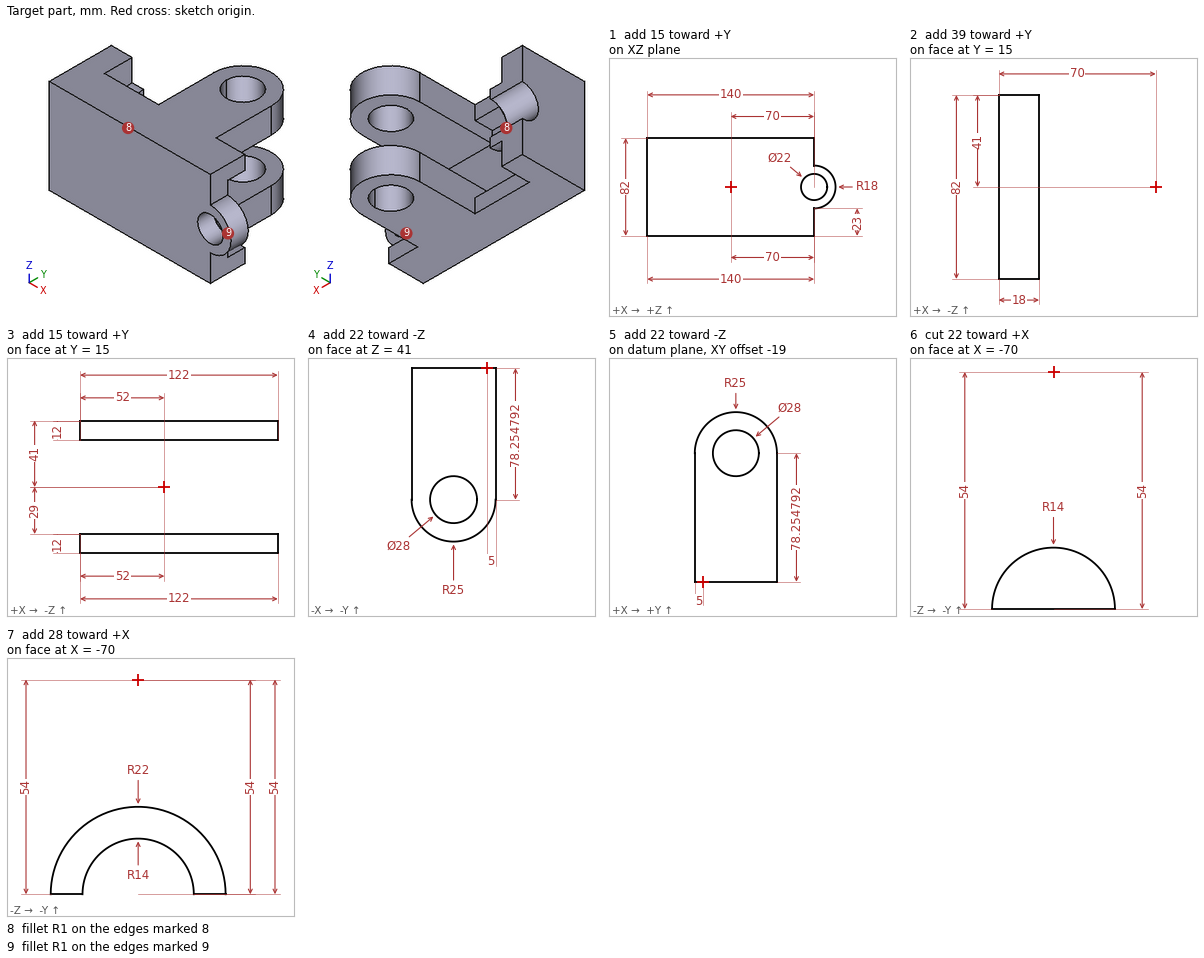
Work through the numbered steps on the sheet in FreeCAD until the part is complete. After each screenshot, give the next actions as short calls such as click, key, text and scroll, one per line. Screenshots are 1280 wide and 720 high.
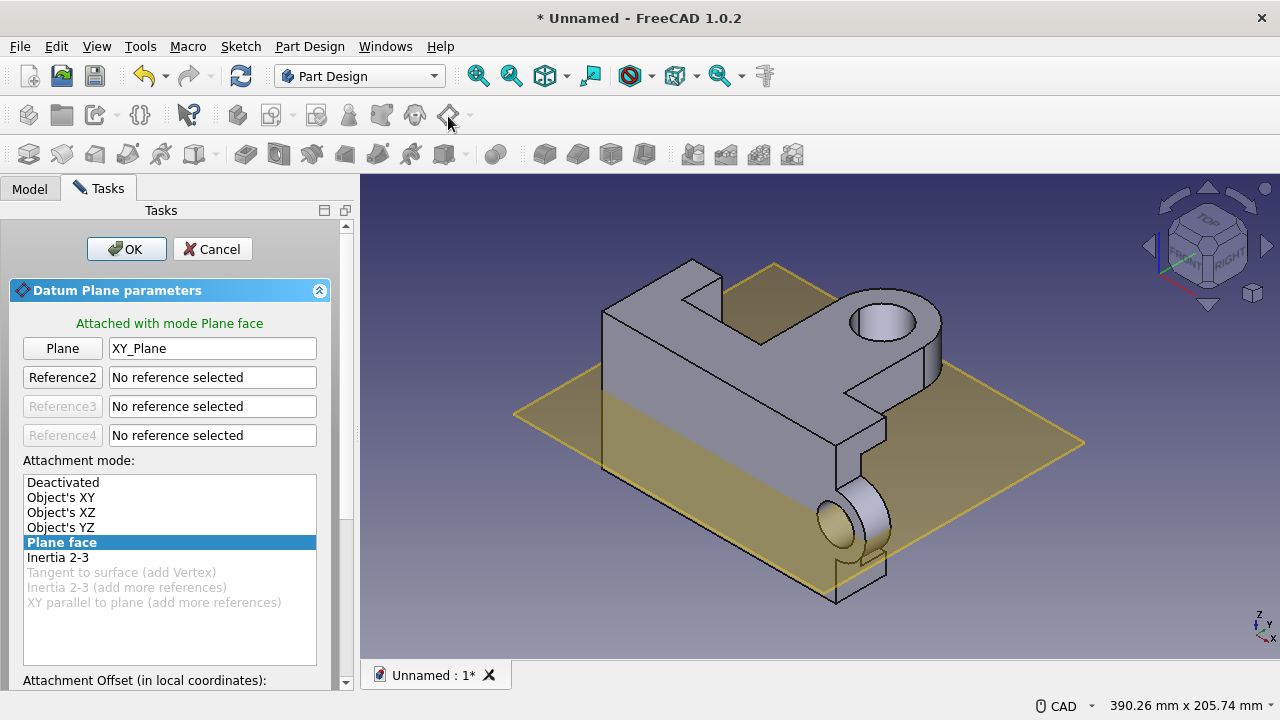
scroll(346, 455, down, 3)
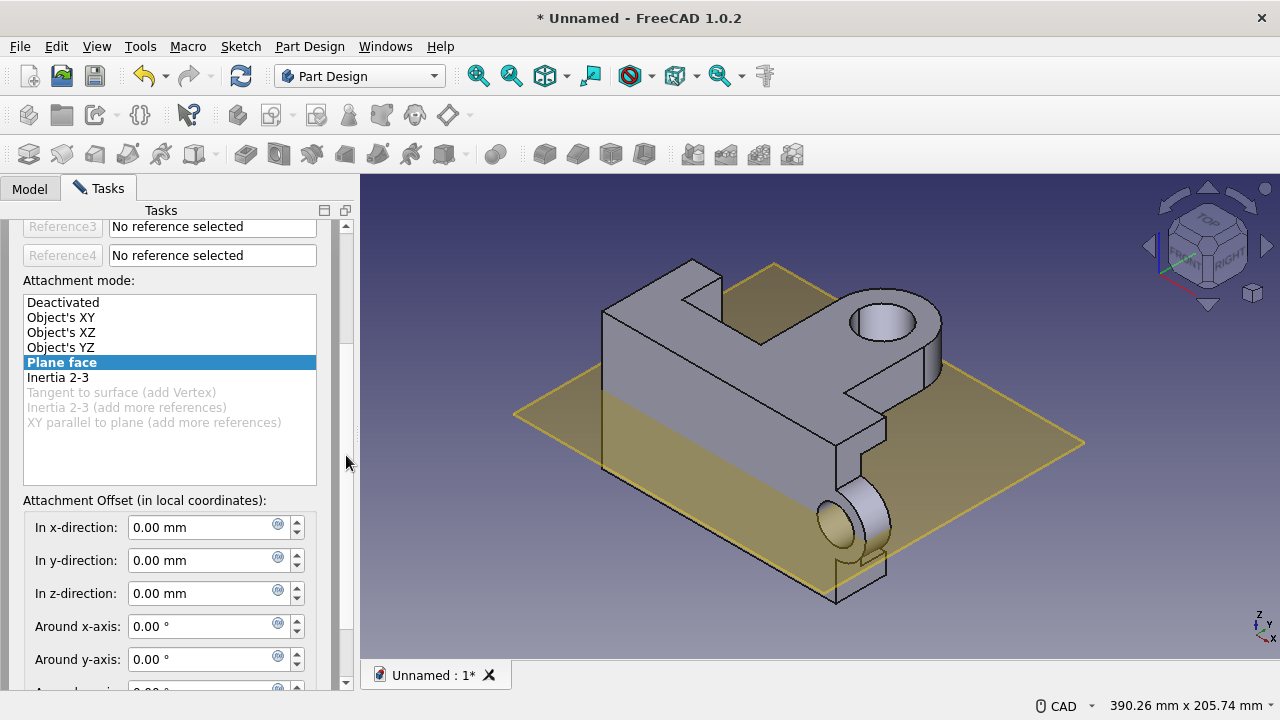
triple_click(210, 594)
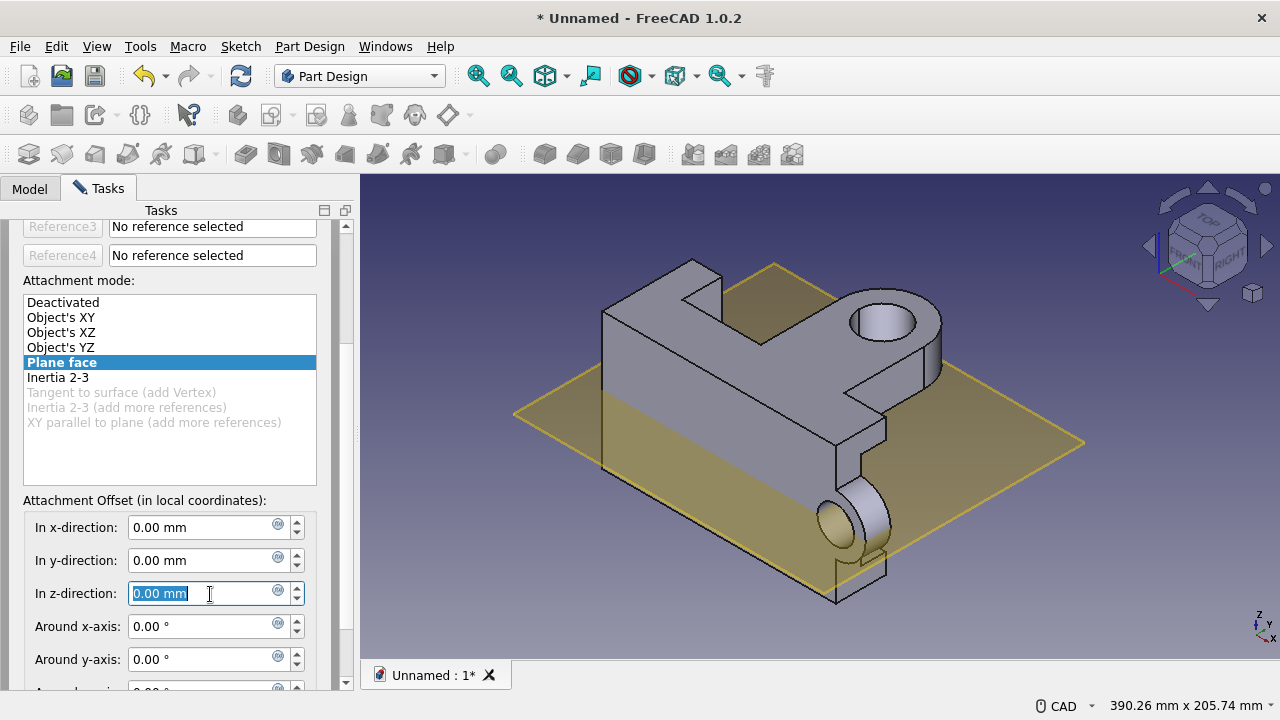
text(-19)
key(Tab)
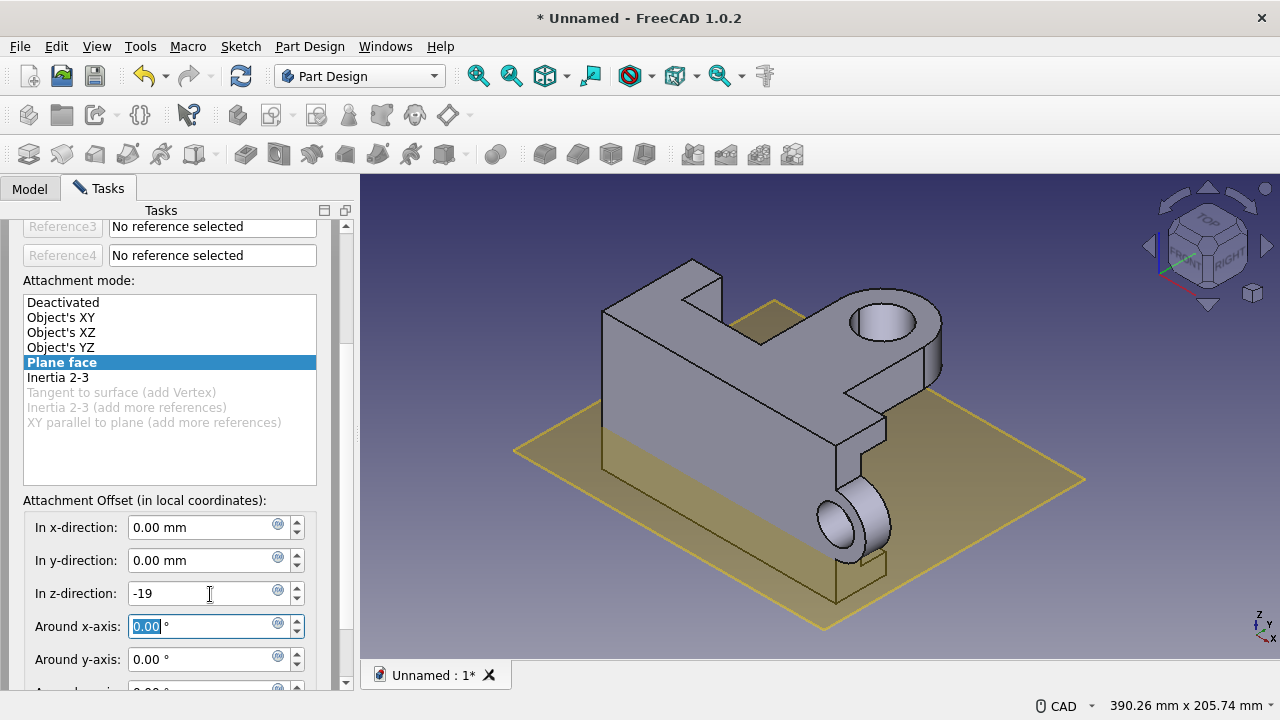
scroll(346, 455, up, 4)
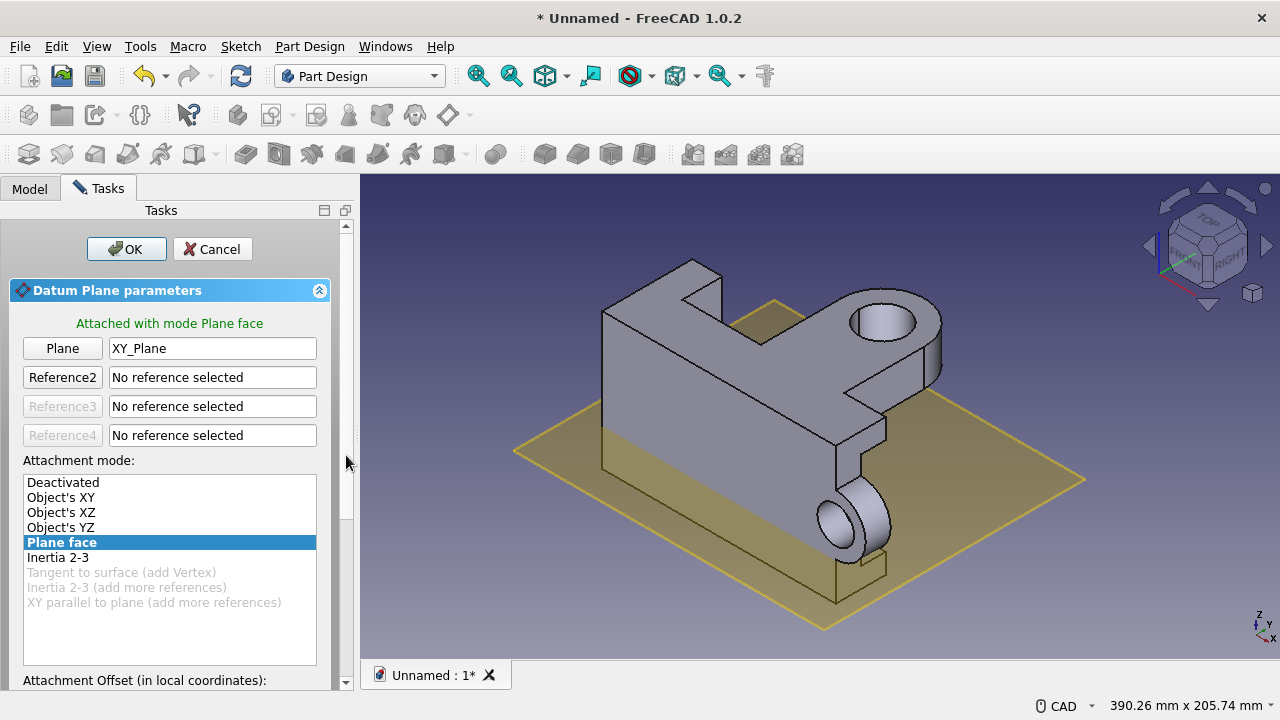
click(127, 249)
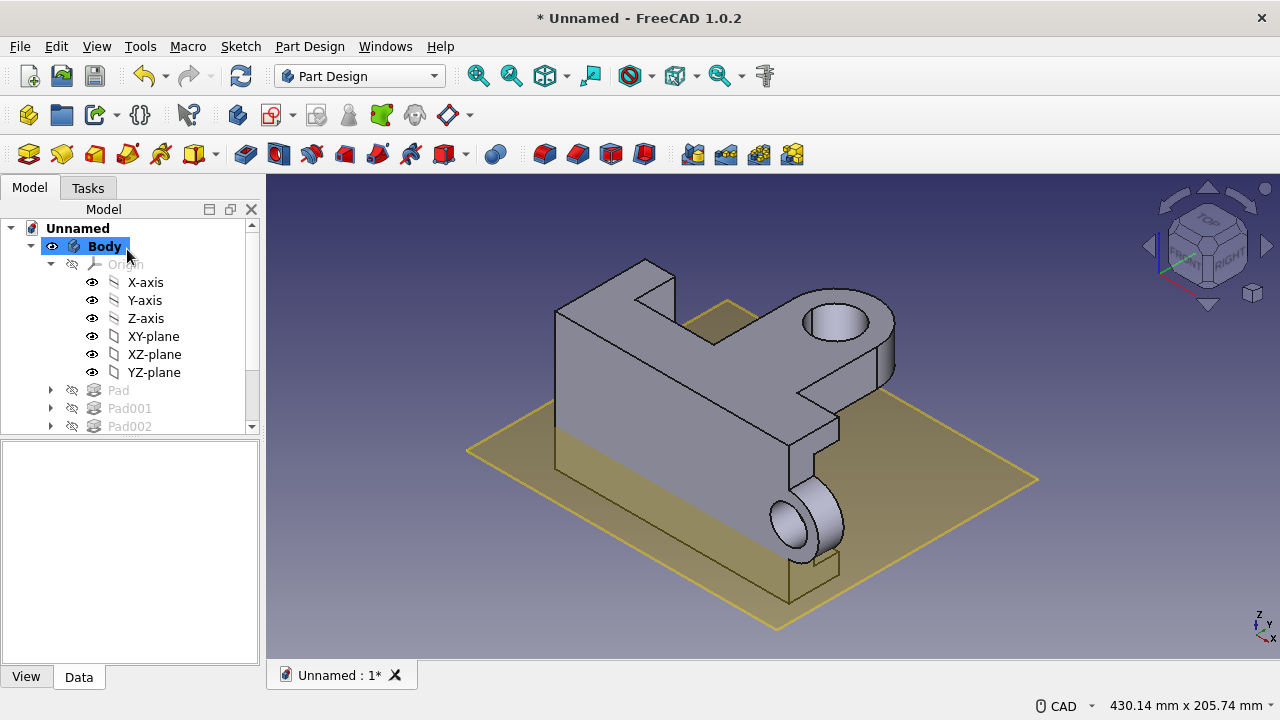
scroll(101, 332, down, 3)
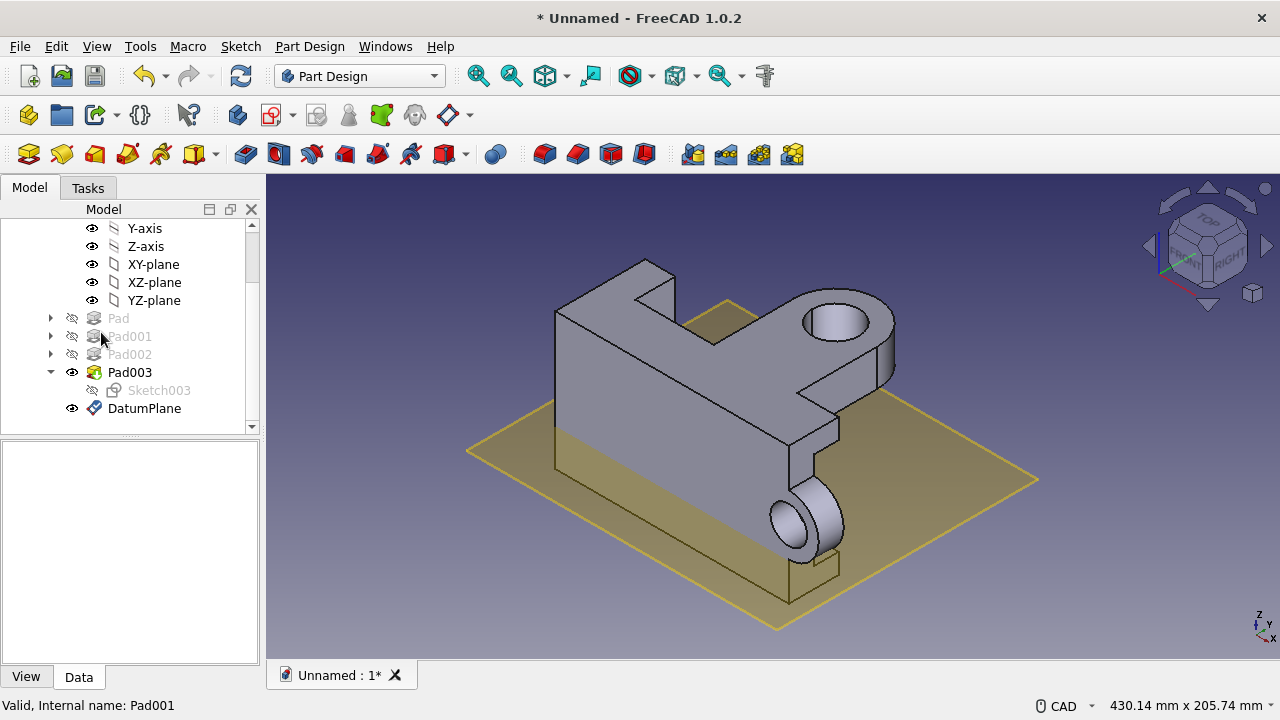
click(117, 408)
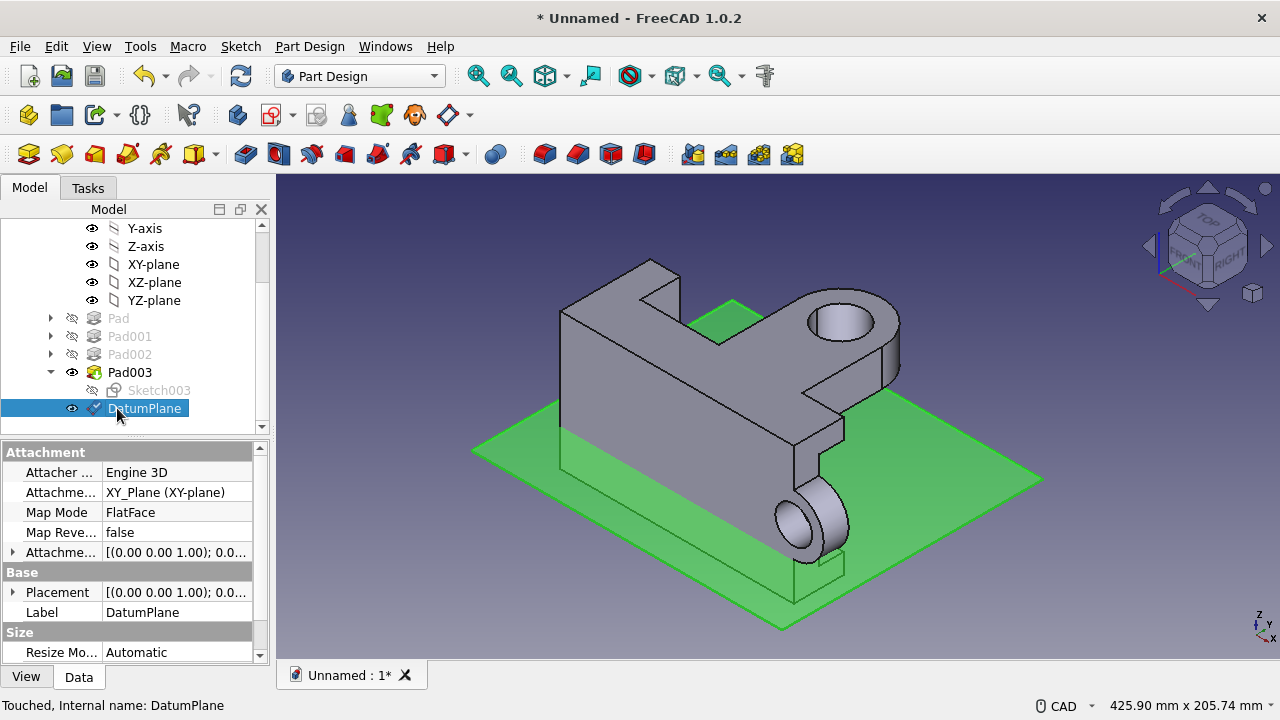
click(270, 116)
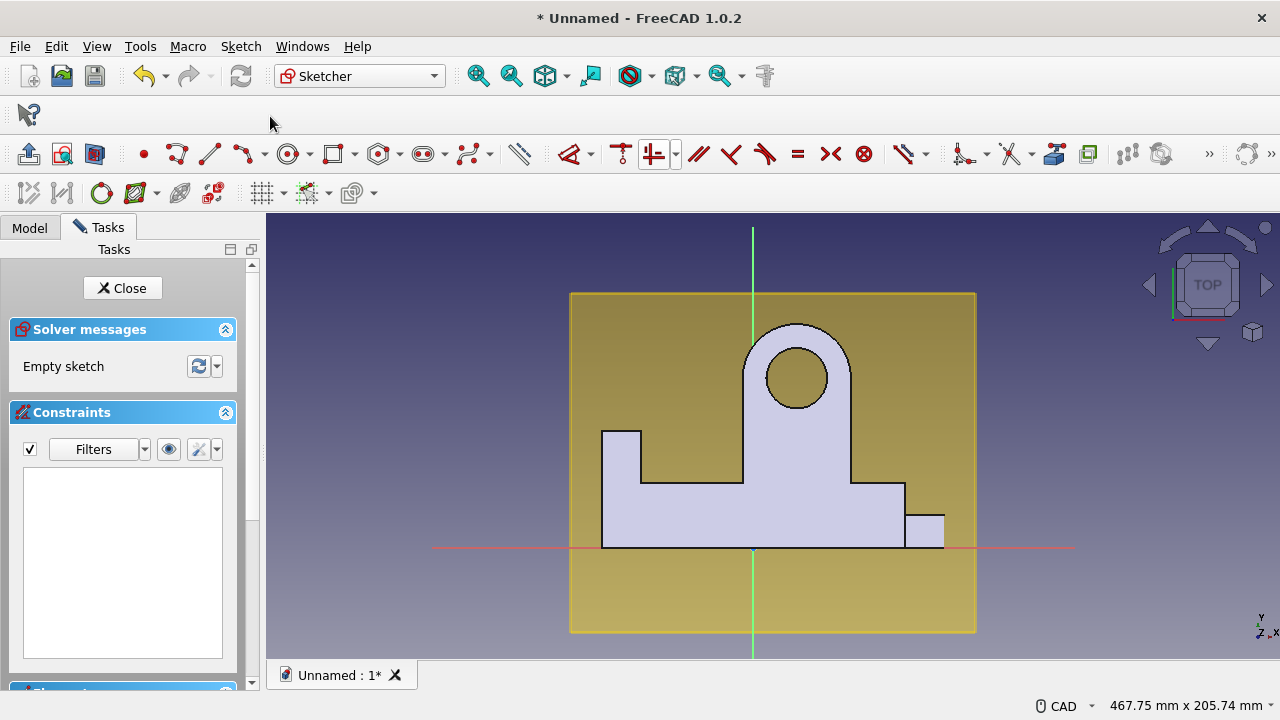
click(95, 154)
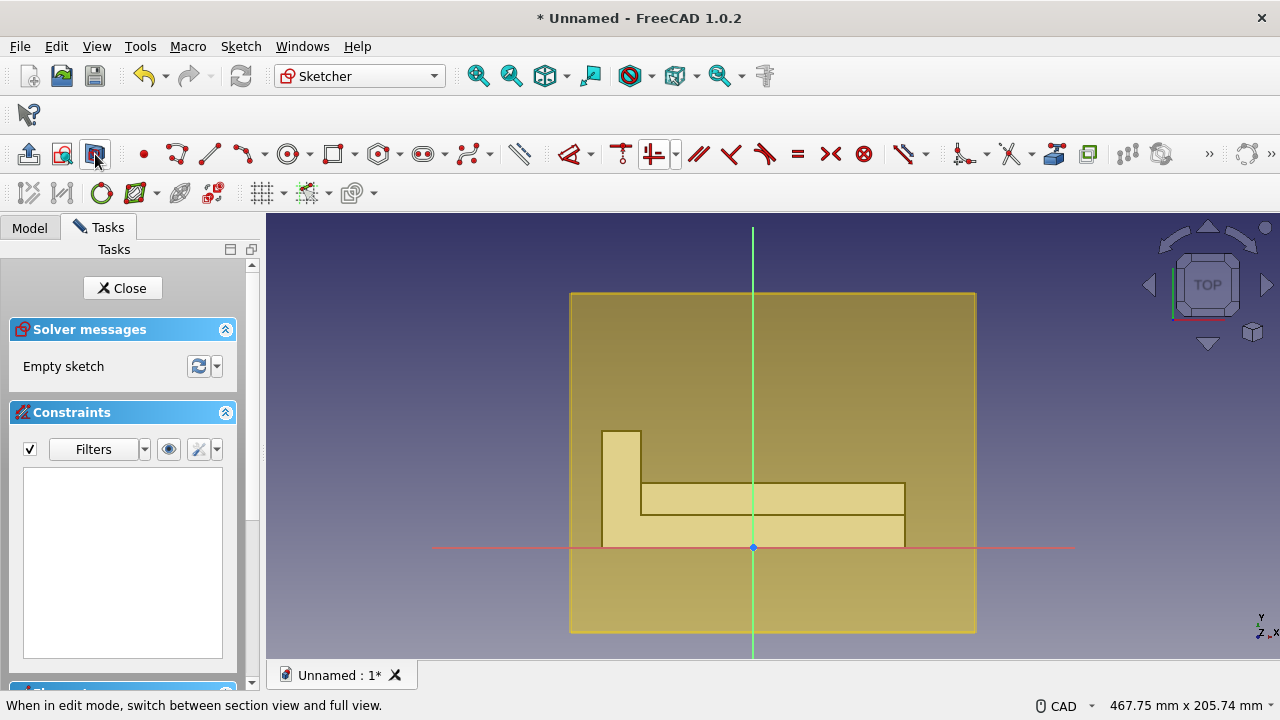
click(177, 154)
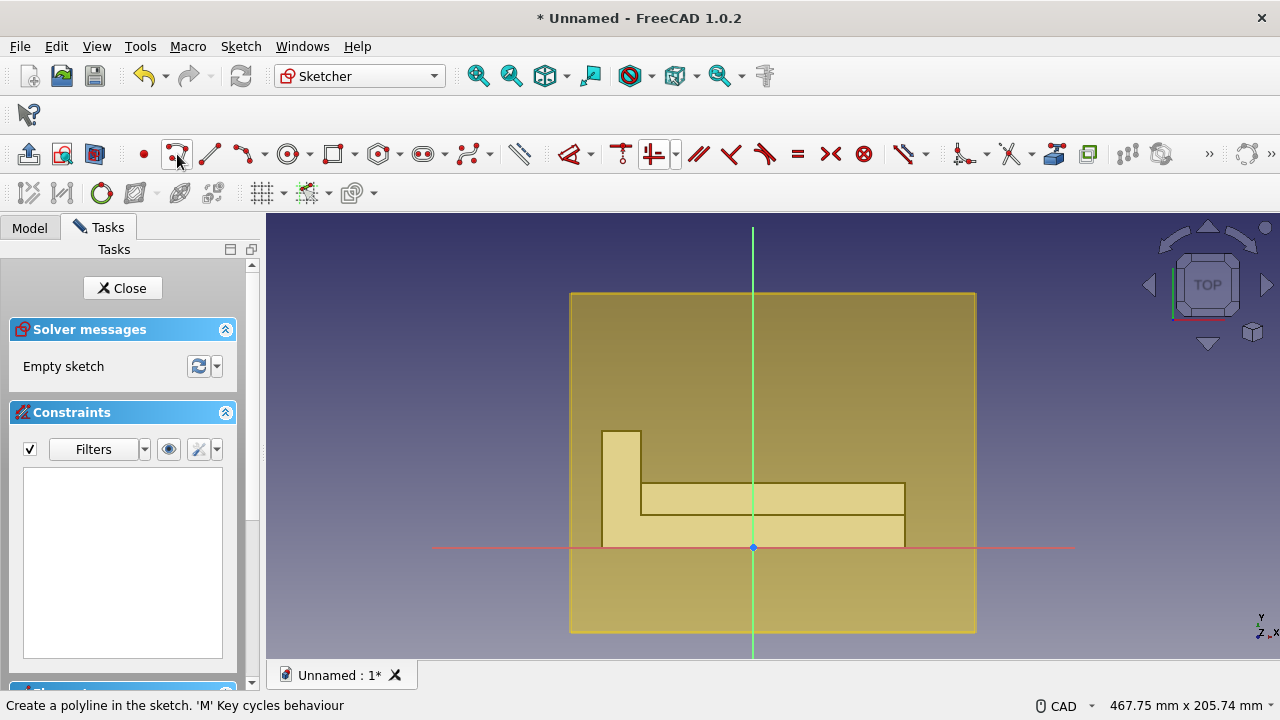
click(851, 378)
click(851, 548)